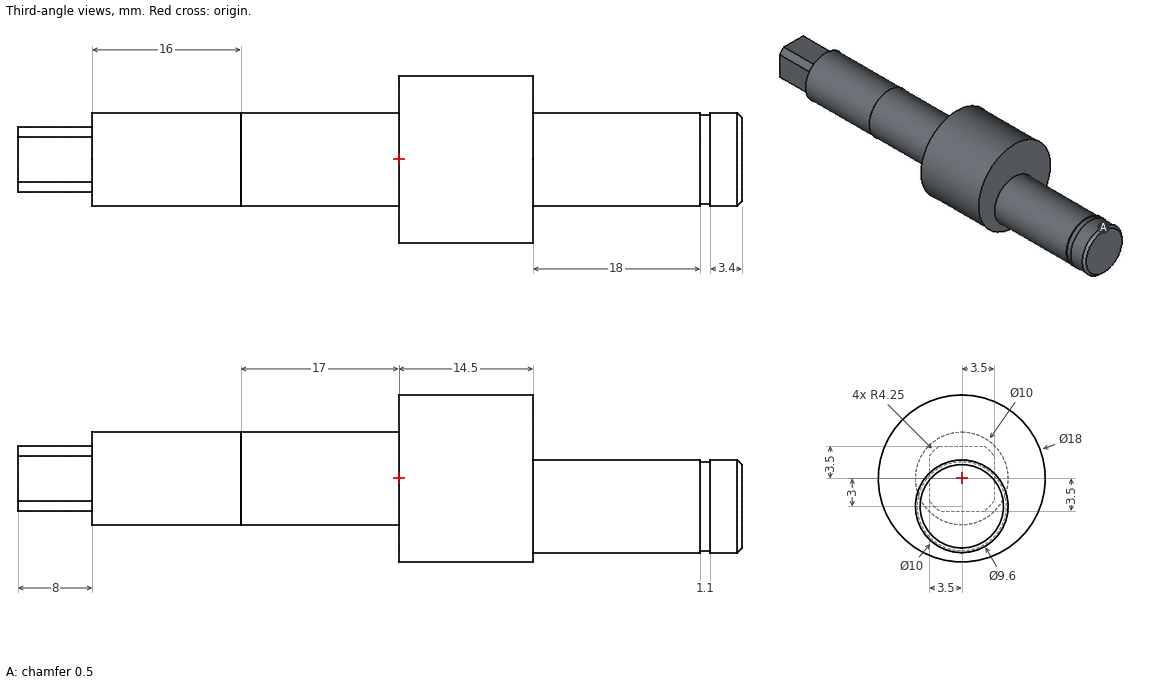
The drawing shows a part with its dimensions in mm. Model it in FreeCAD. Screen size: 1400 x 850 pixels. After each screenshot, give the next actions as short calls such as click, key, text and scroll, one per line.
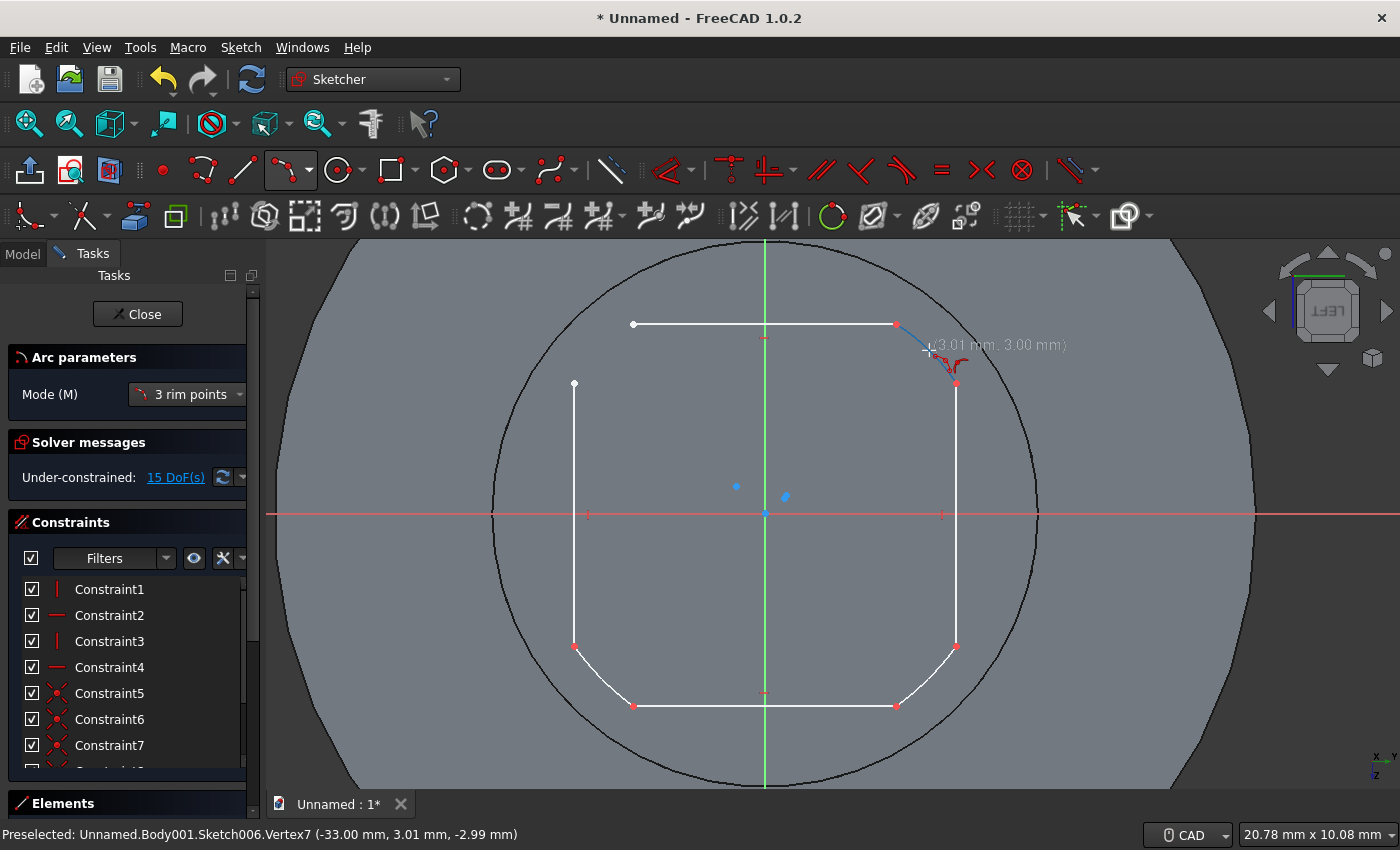
click(633, 324)
click(574, 383)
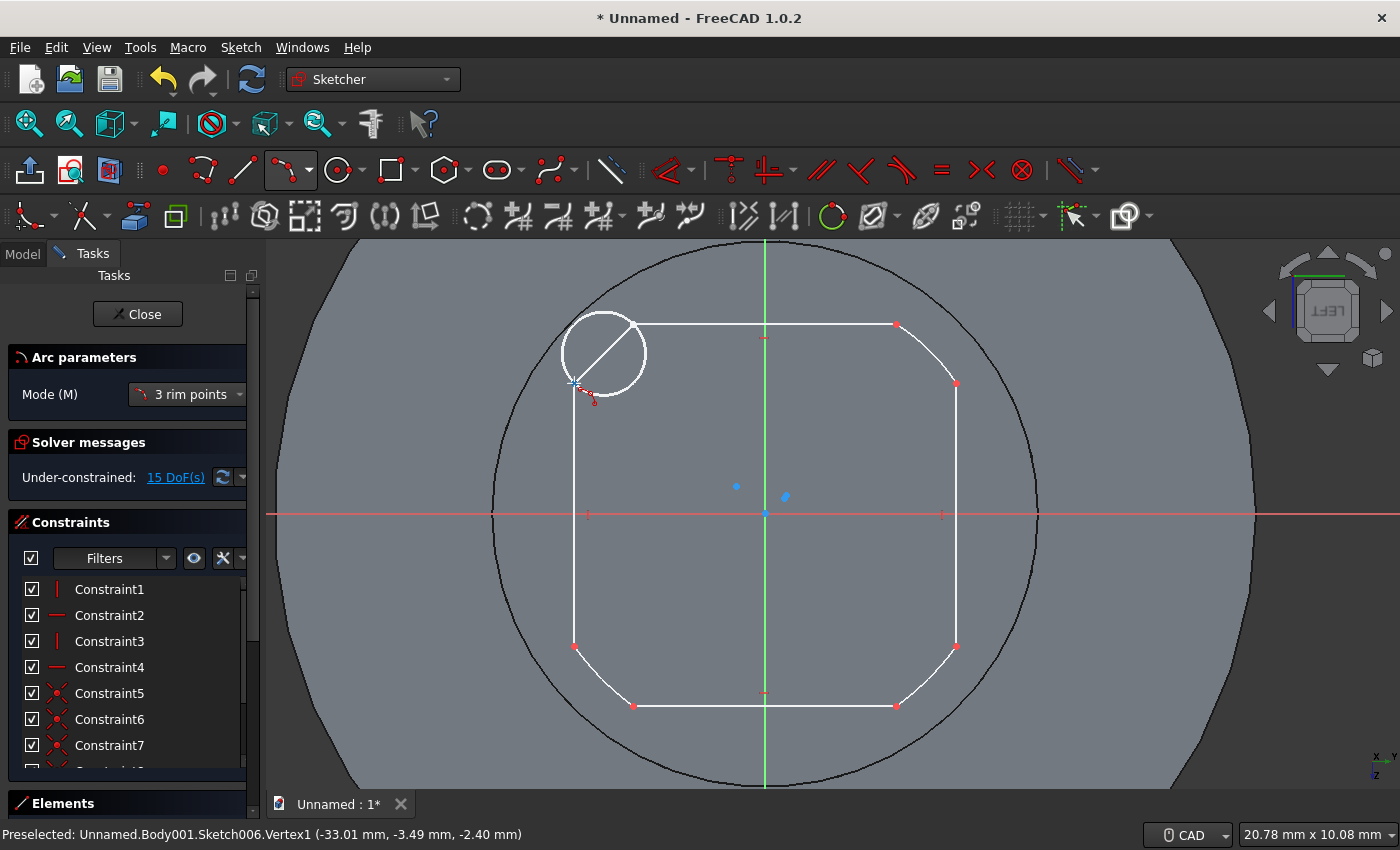
scroll(601, 350, up, 8)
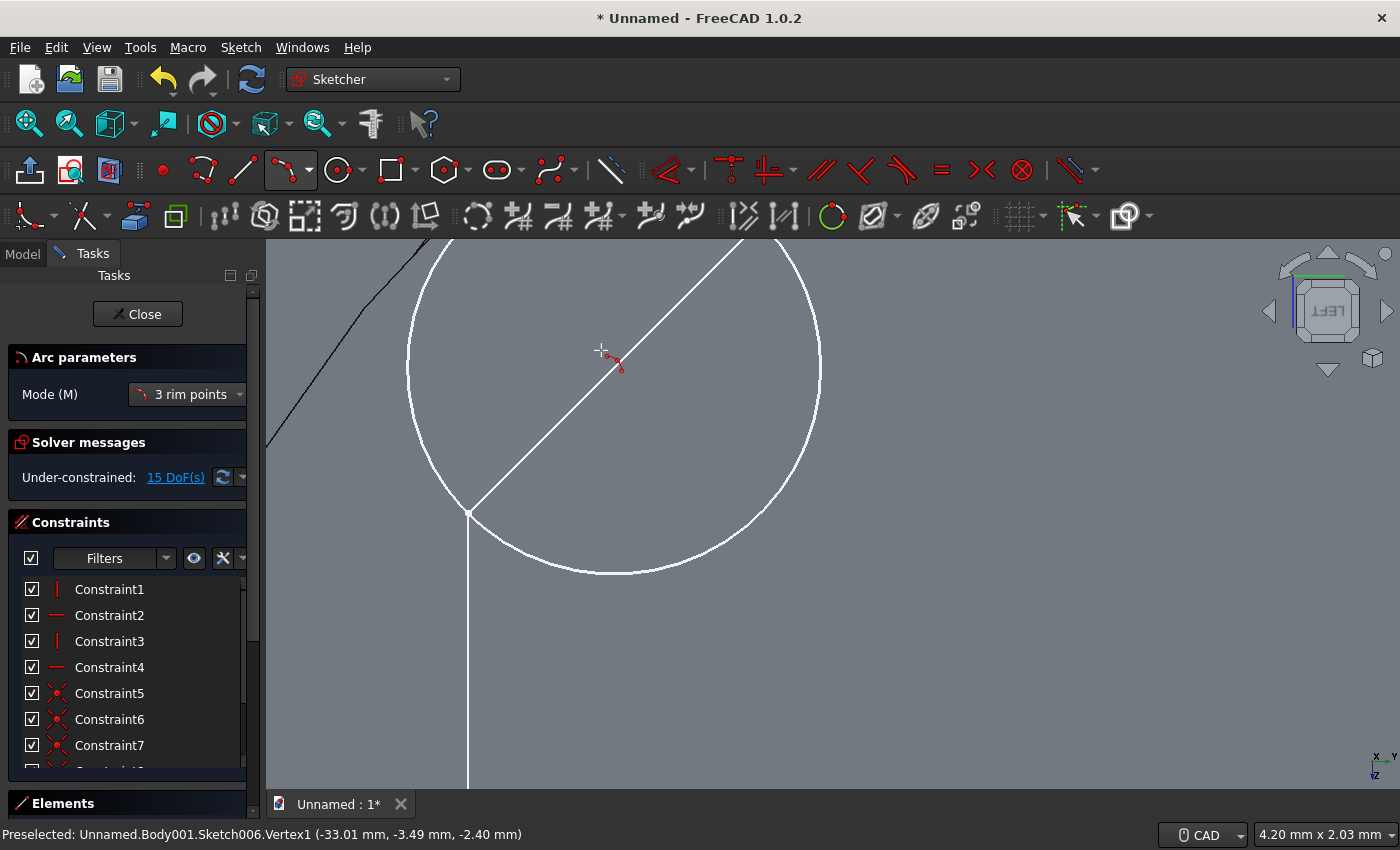
click(600, 349)
key(Escape)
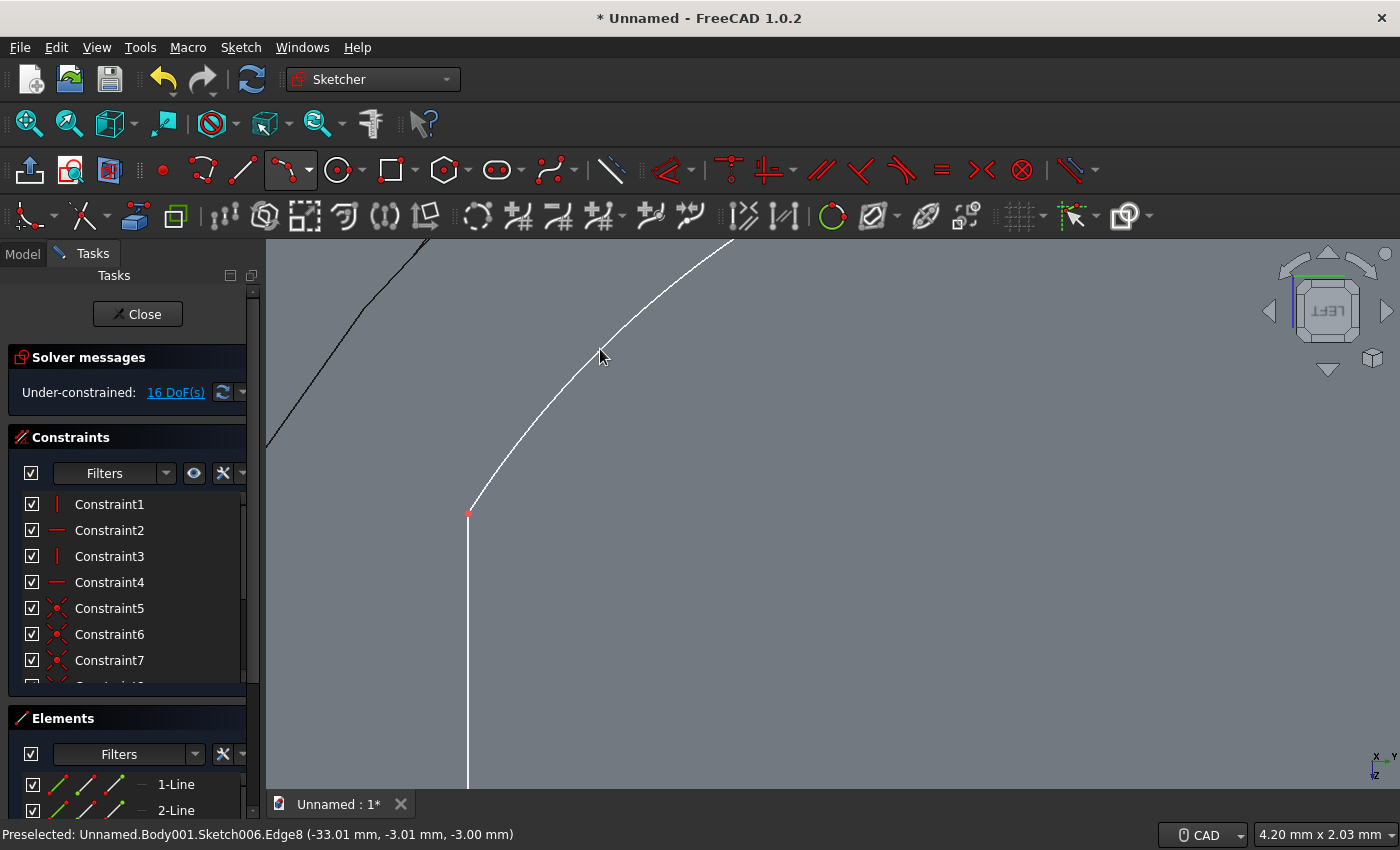
scroll(601, 350, down, 8)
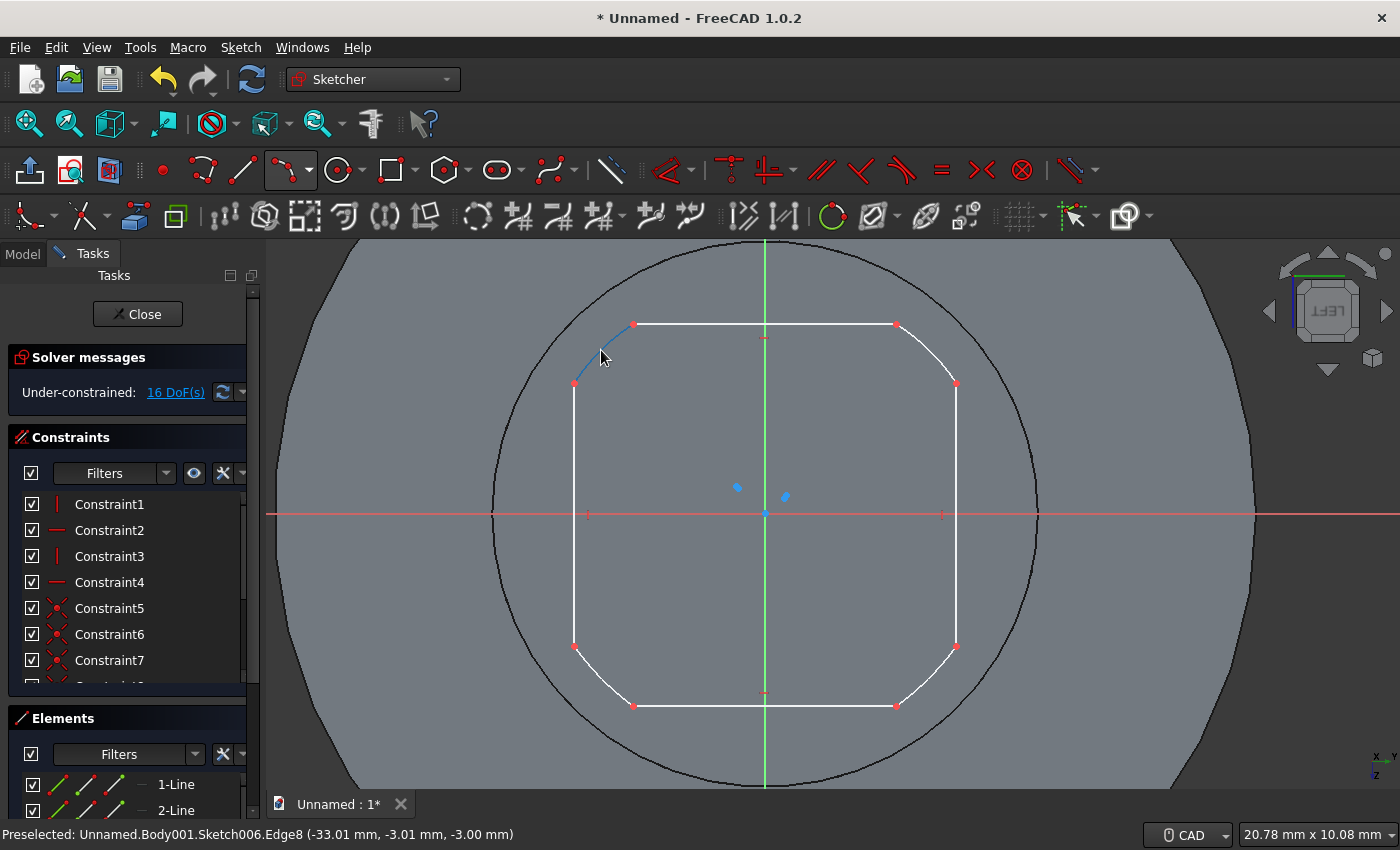
click(590, 666)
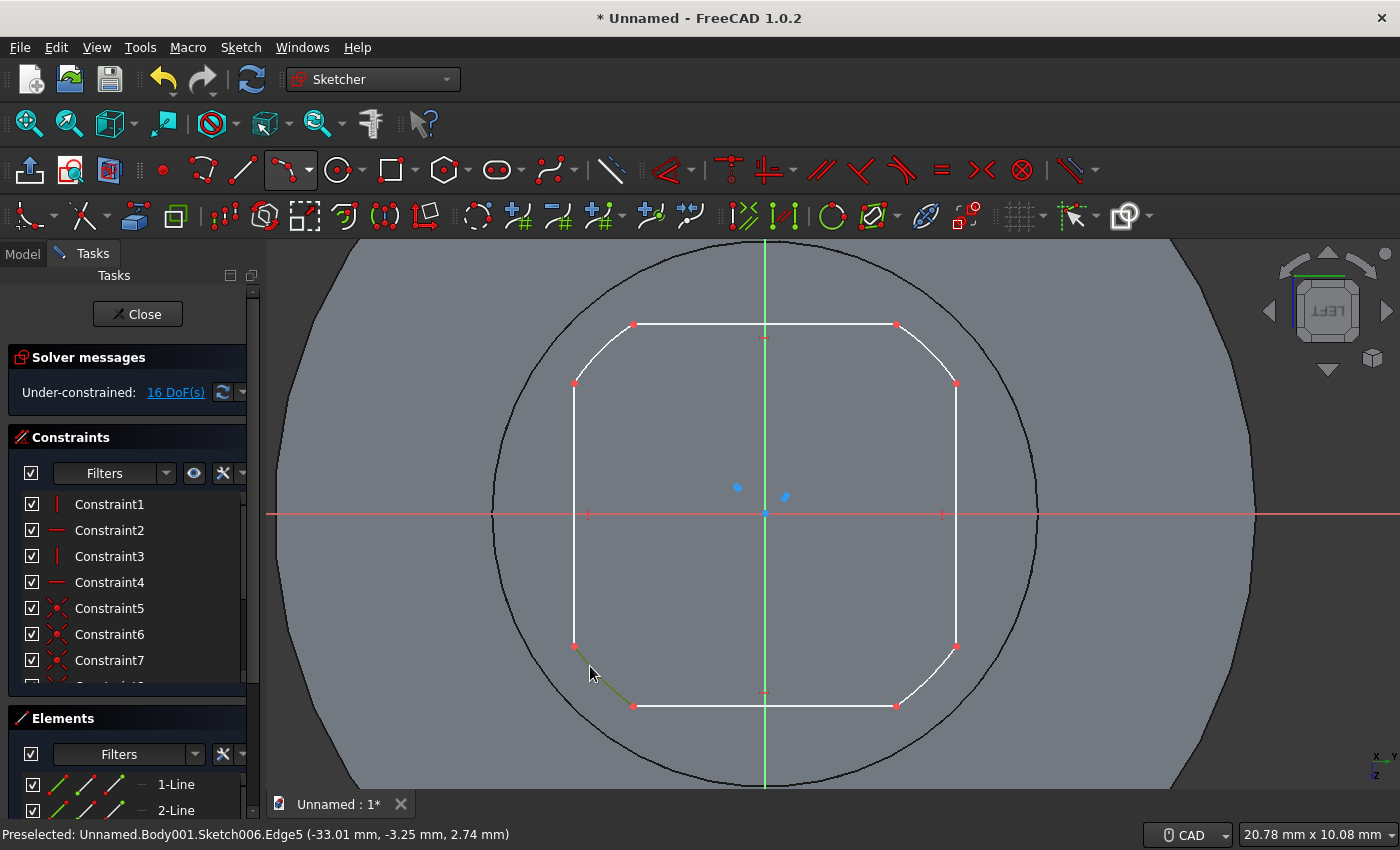
click(916, 690)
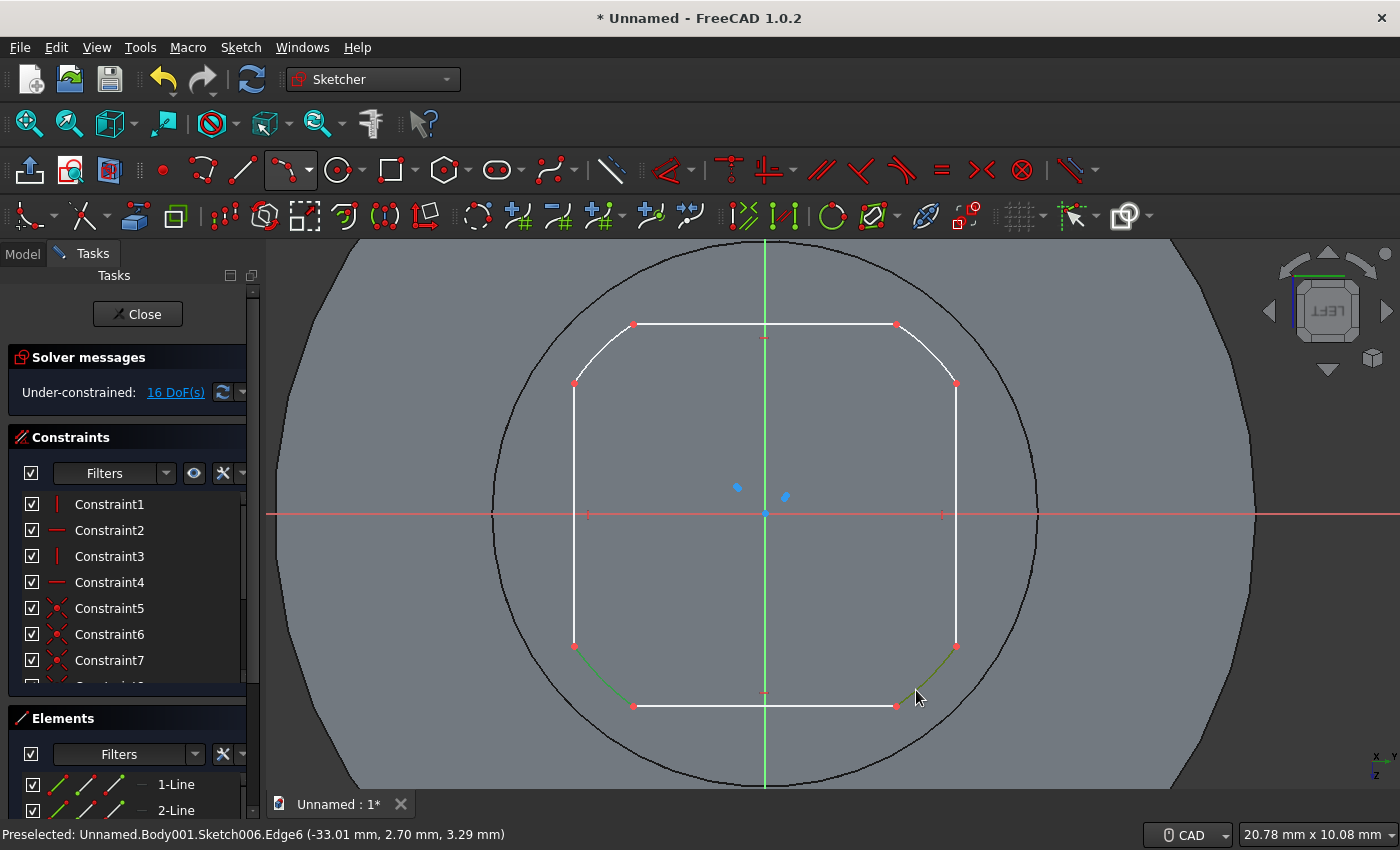
click(730, 170)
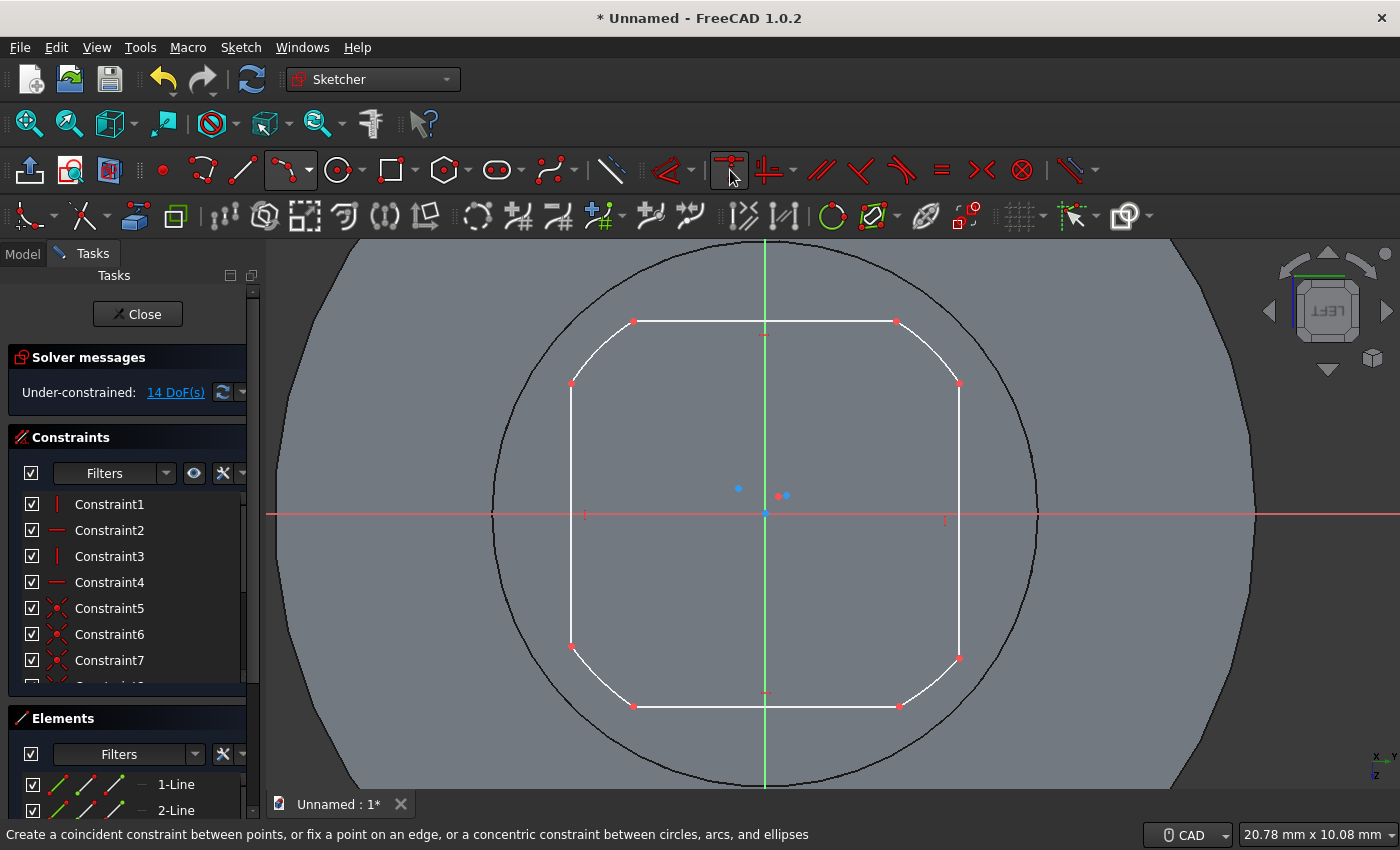
click(588, 666)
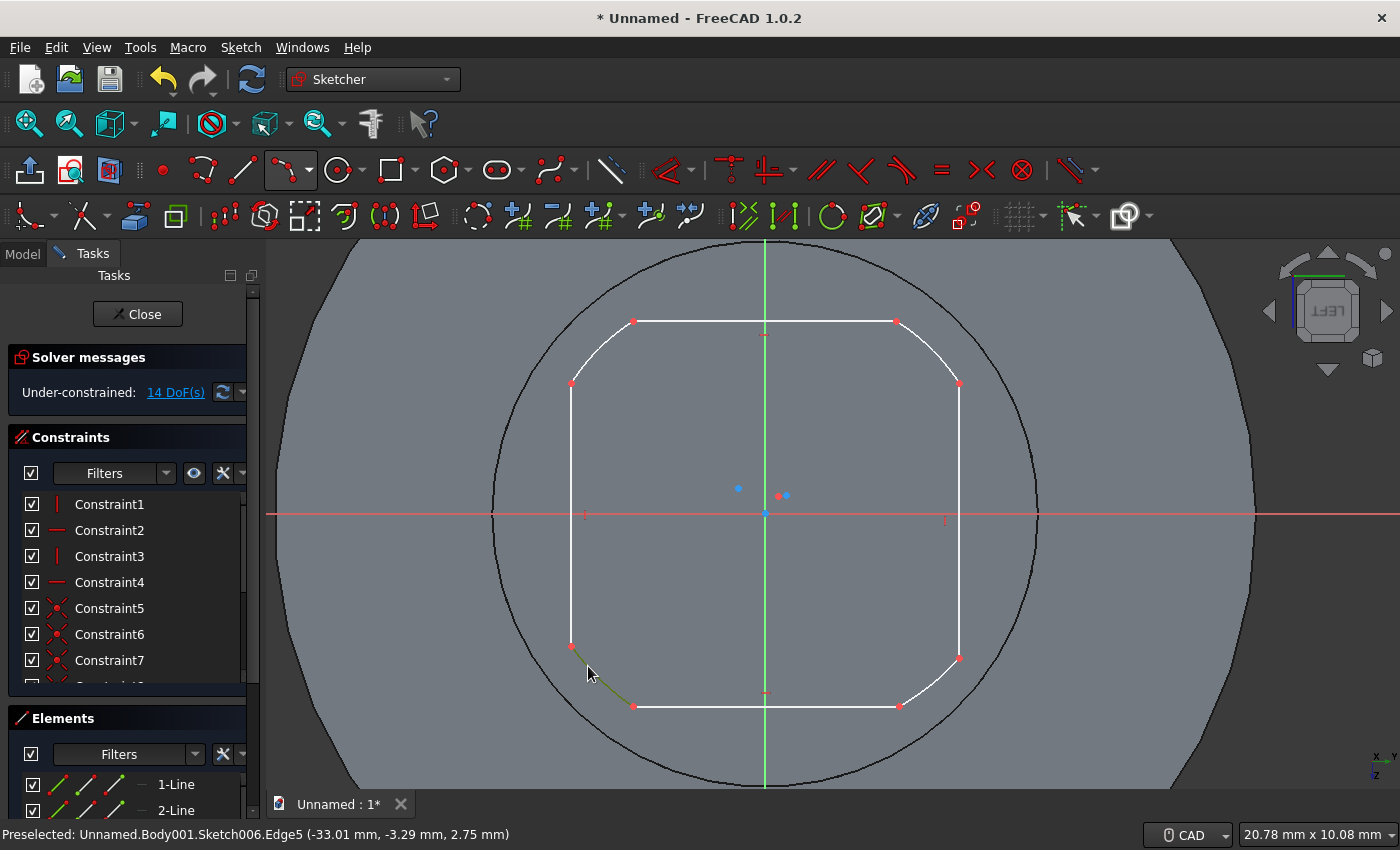
click(943, 362)